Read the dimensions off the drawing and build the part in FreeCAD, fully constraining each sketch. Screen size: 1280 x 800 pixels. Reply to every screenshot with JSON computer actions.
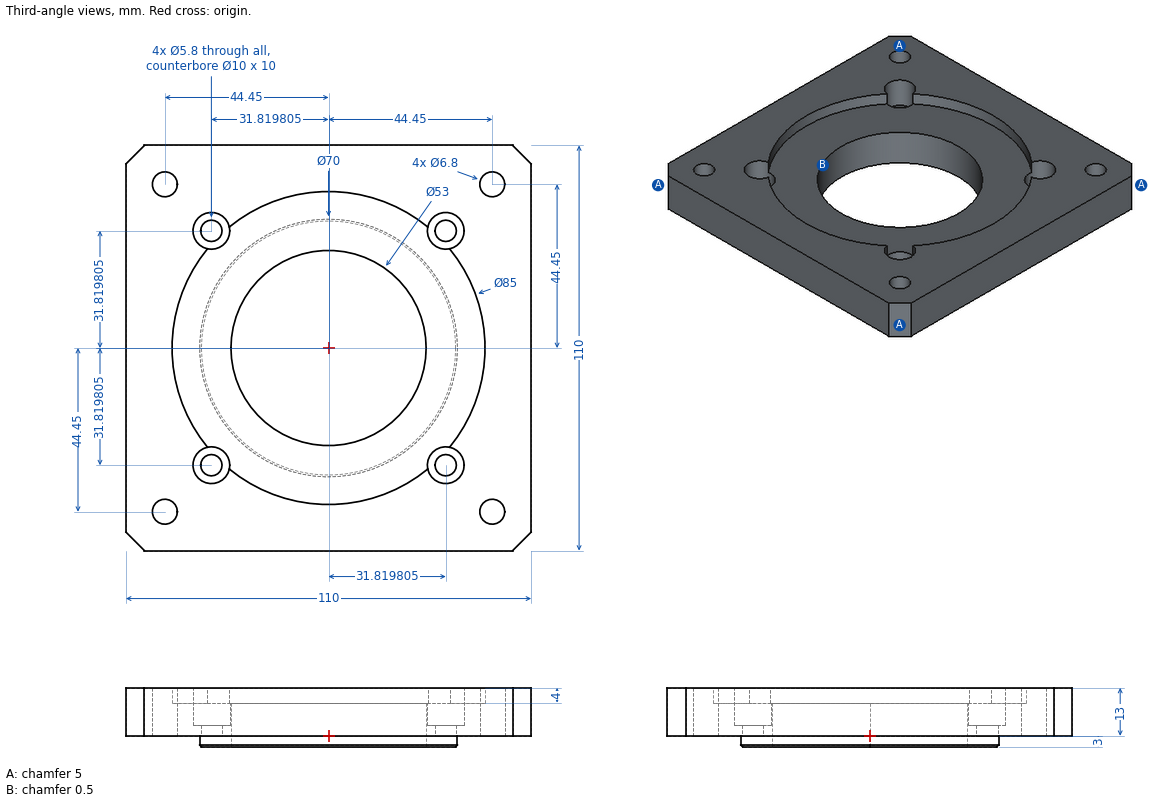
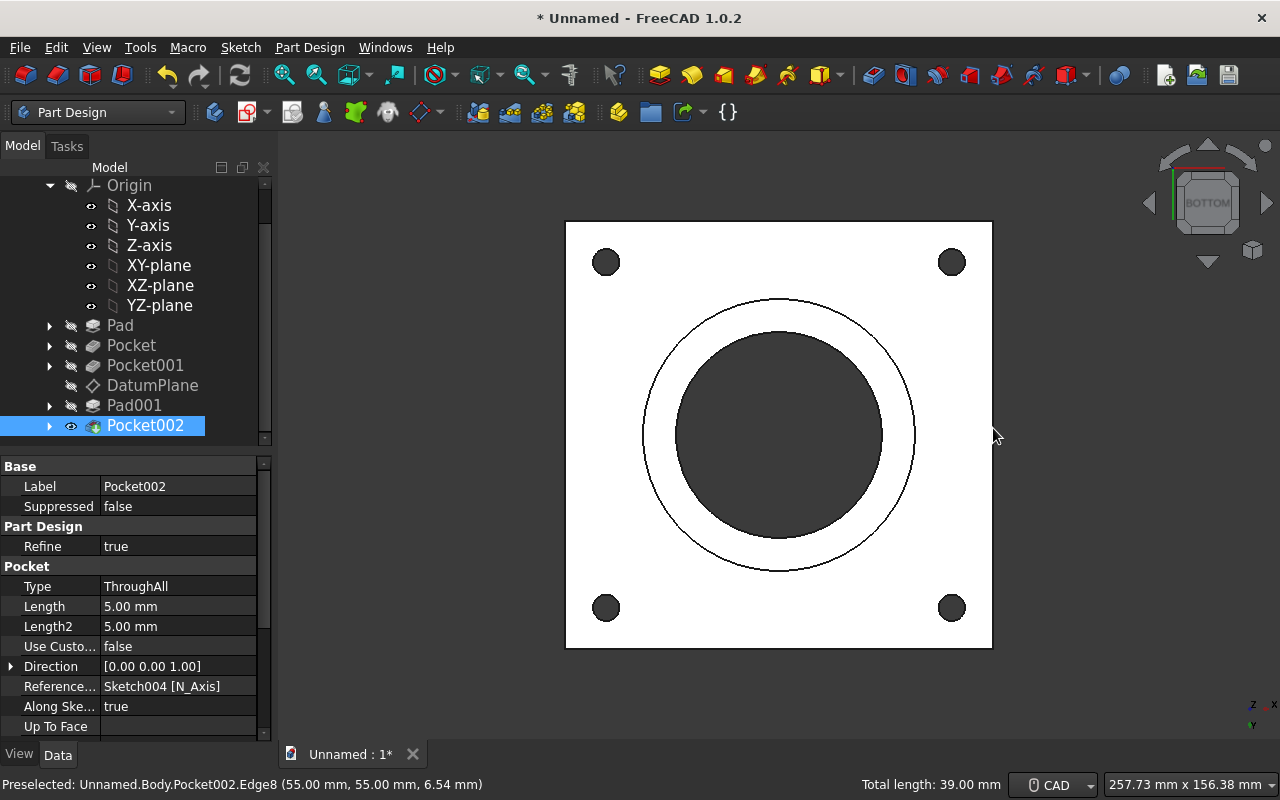
{"action": "key", "text": "4"}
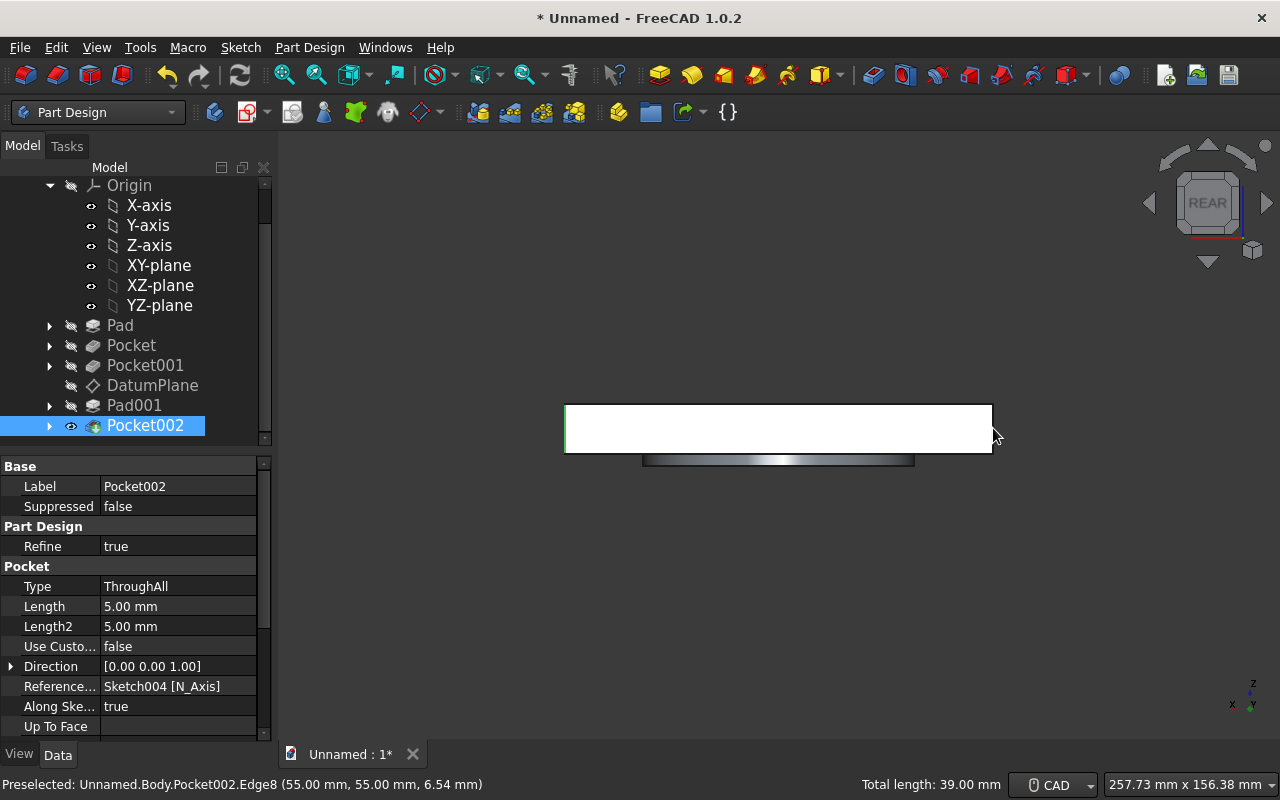
{"action": "left_click", "coordinate": [286, 76]}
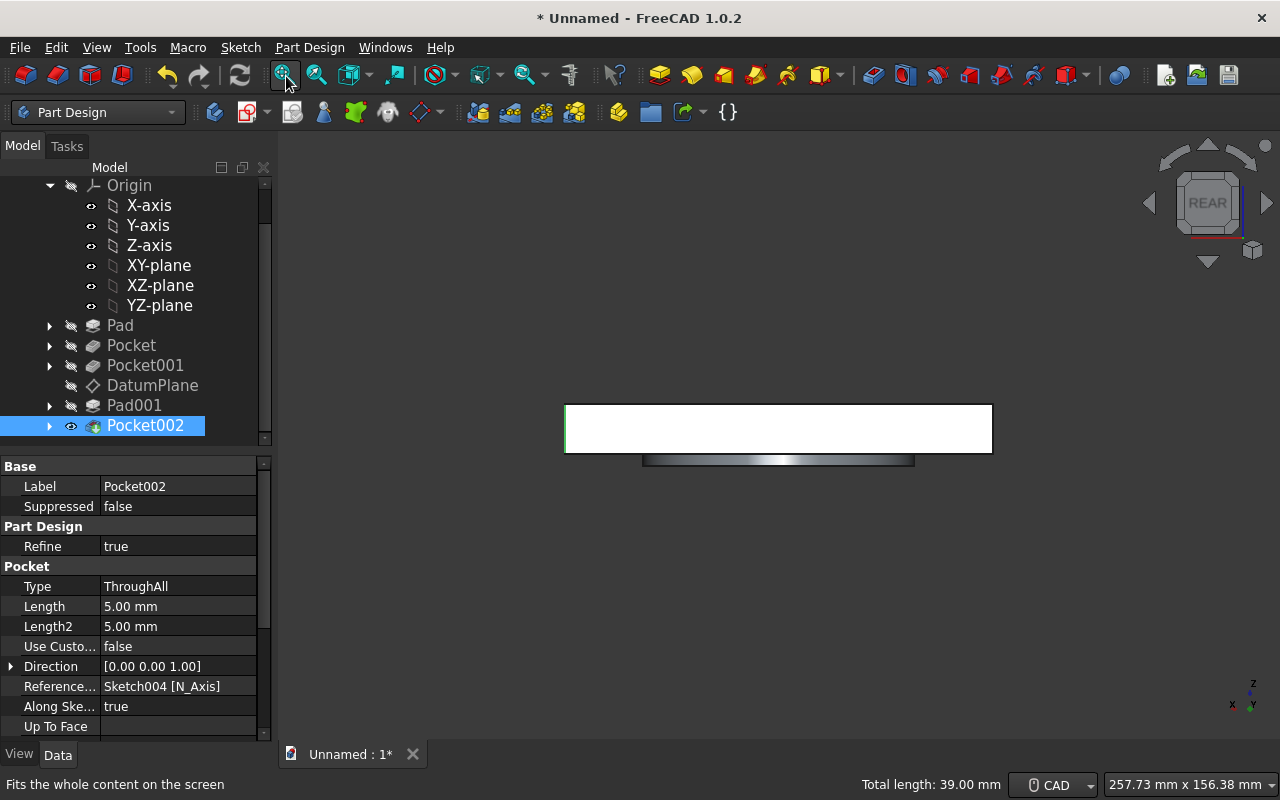
{"action": "left_click", "coordinate": [993, 428], "text": "ctrl"}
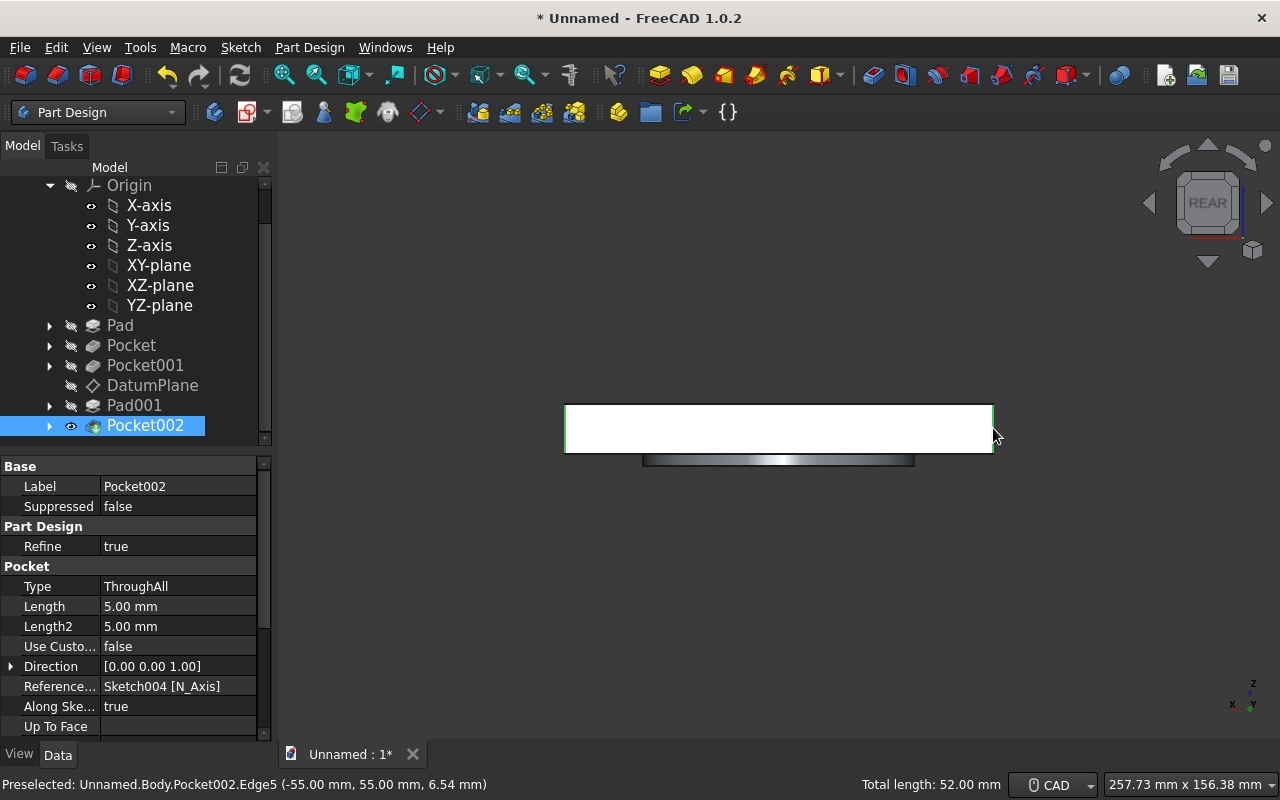
{"action": "left_click", "coordinate": [58, 76]}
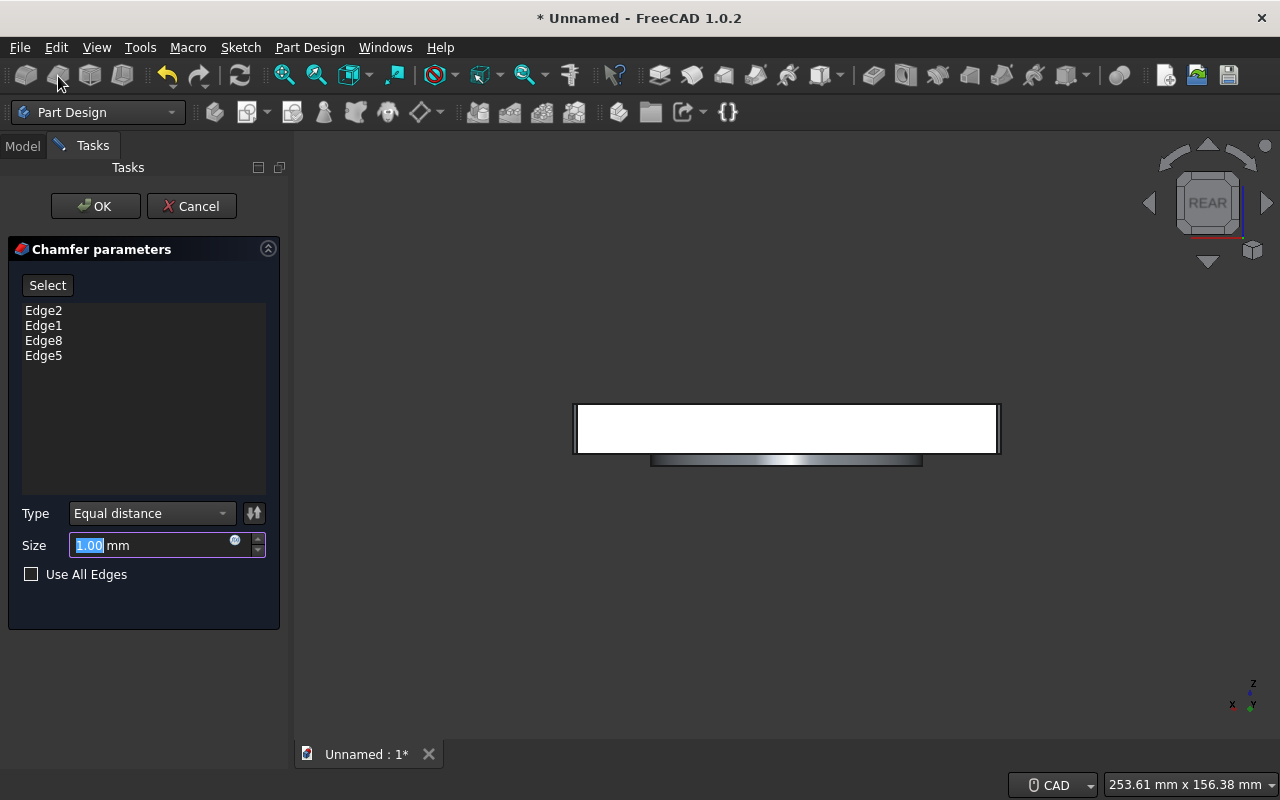
{"action": "type", "text": "5"}
{"action": "key", "text": "Tab"}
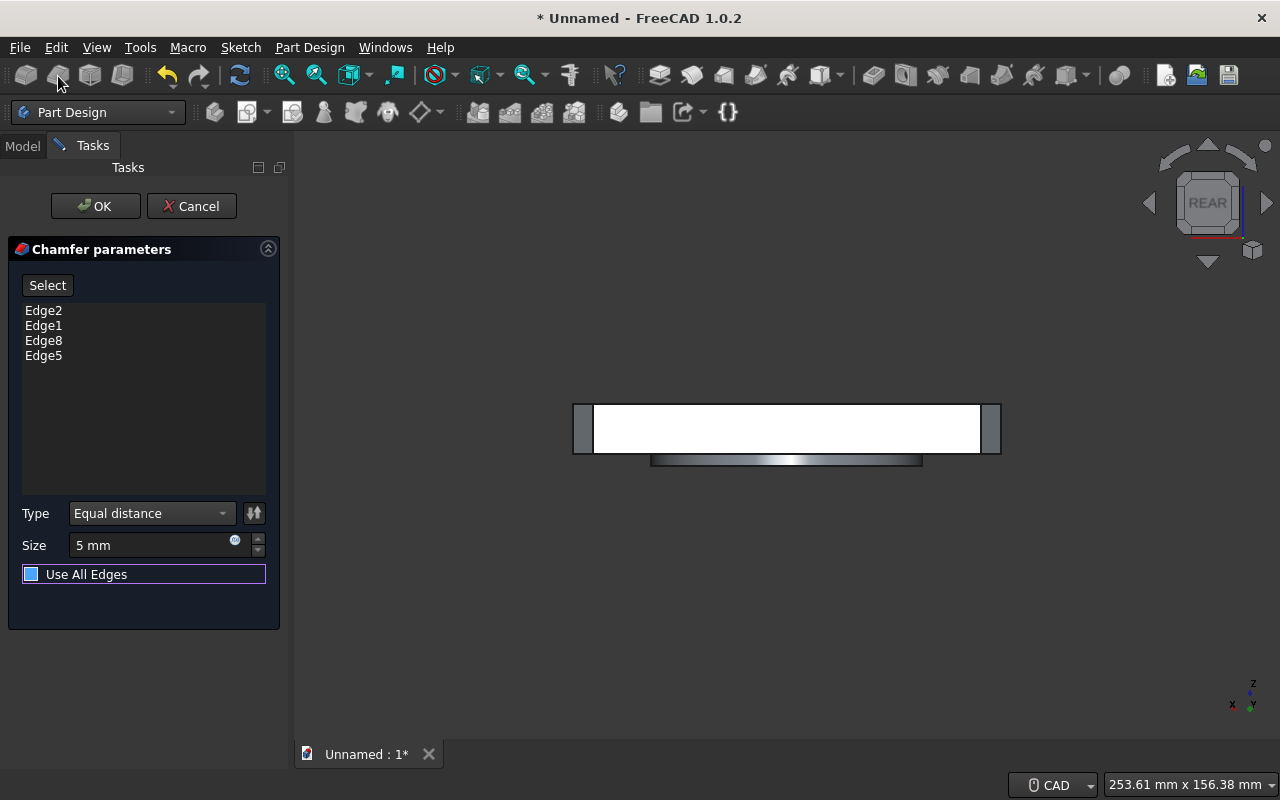
{"action": "left_click", "coordinate": [96, 206]}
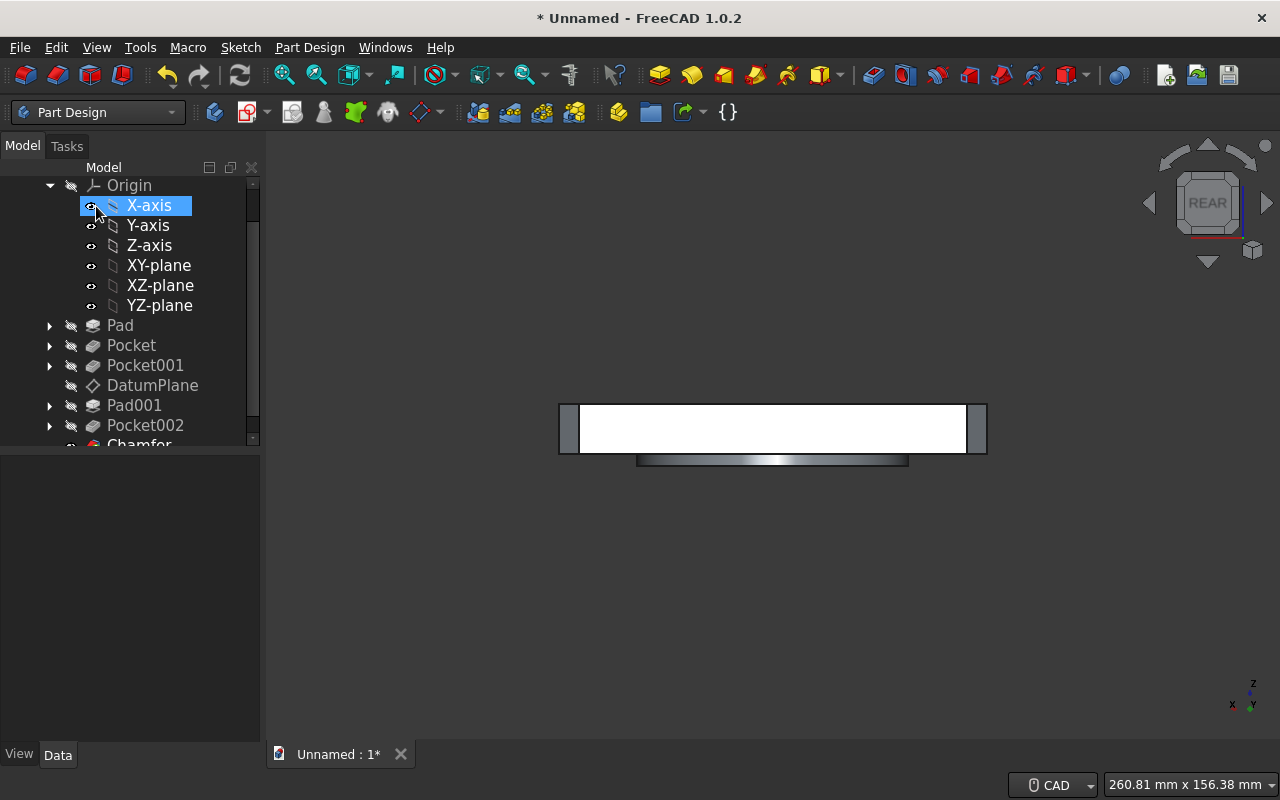
{"action": "key", "text": "v f"}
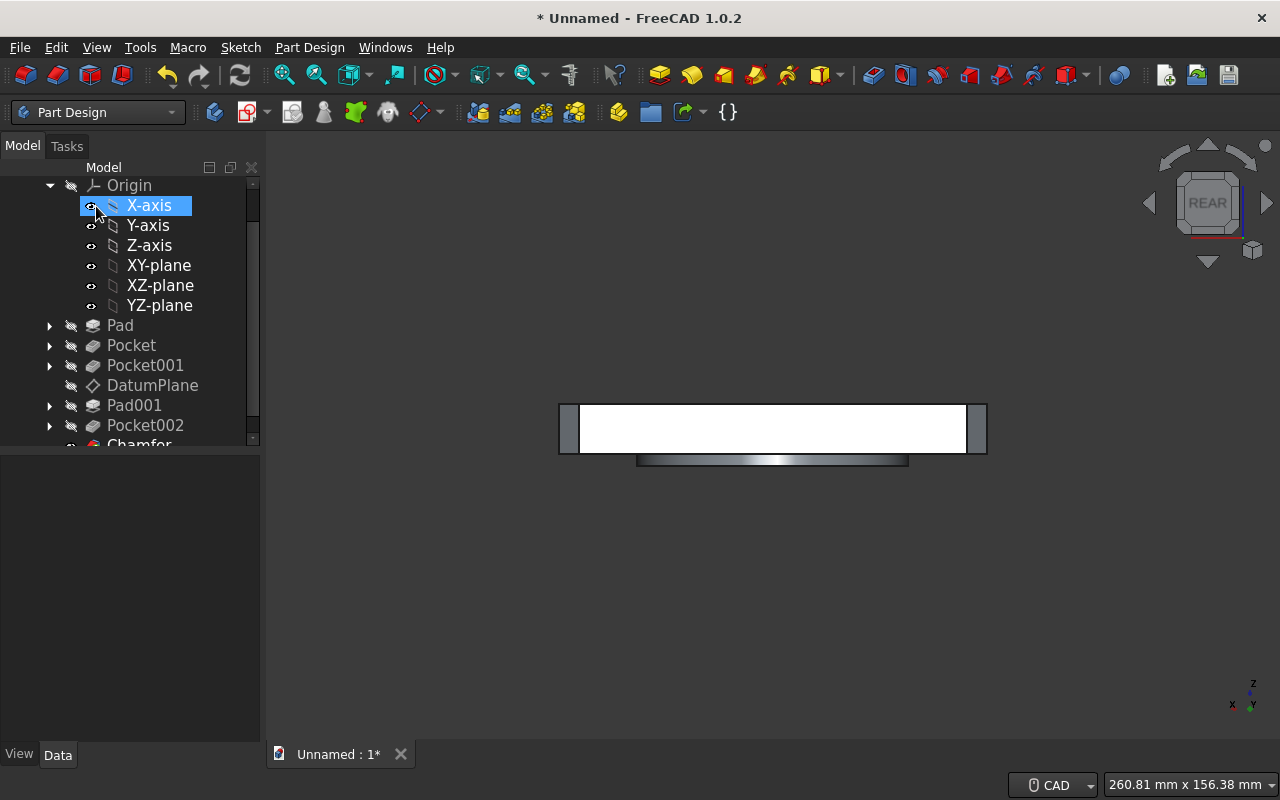
{"action": "key", "text": "0"}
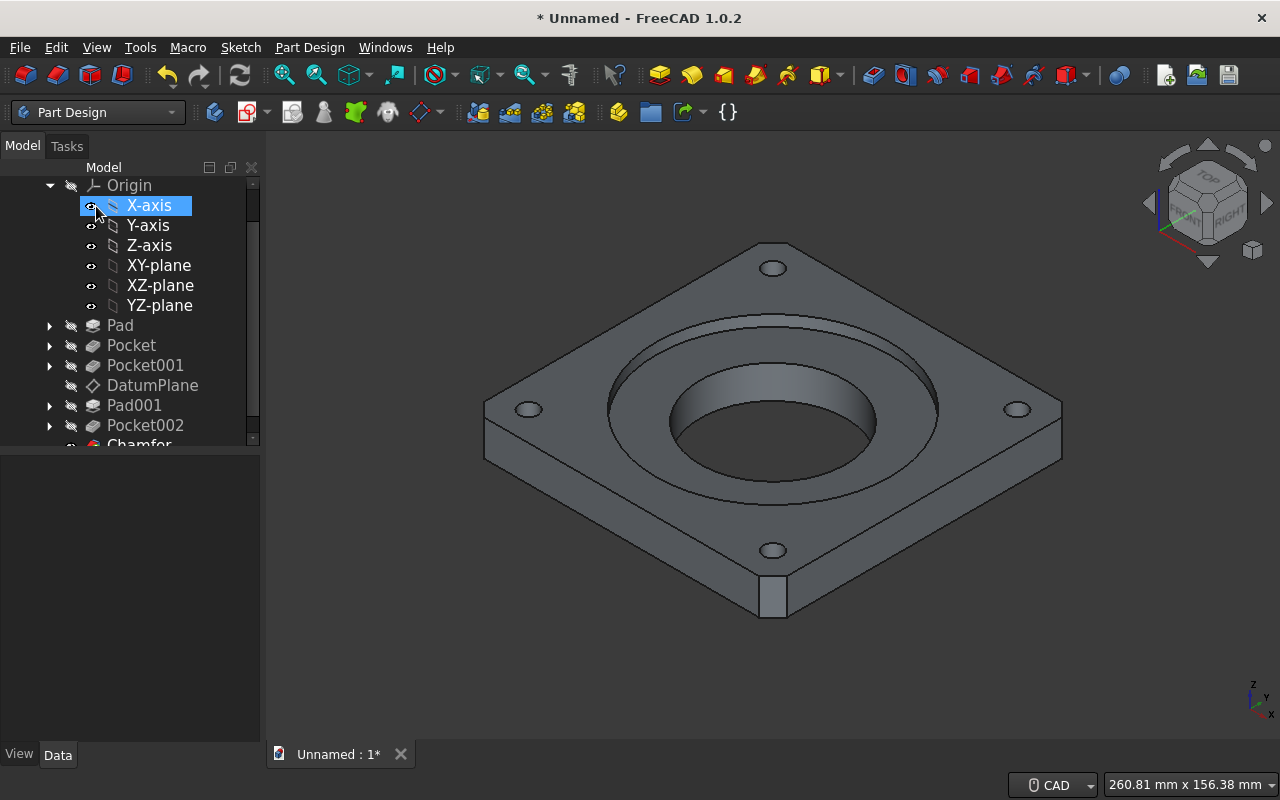
{"action": "left_click", "coordinate": [989, 434]}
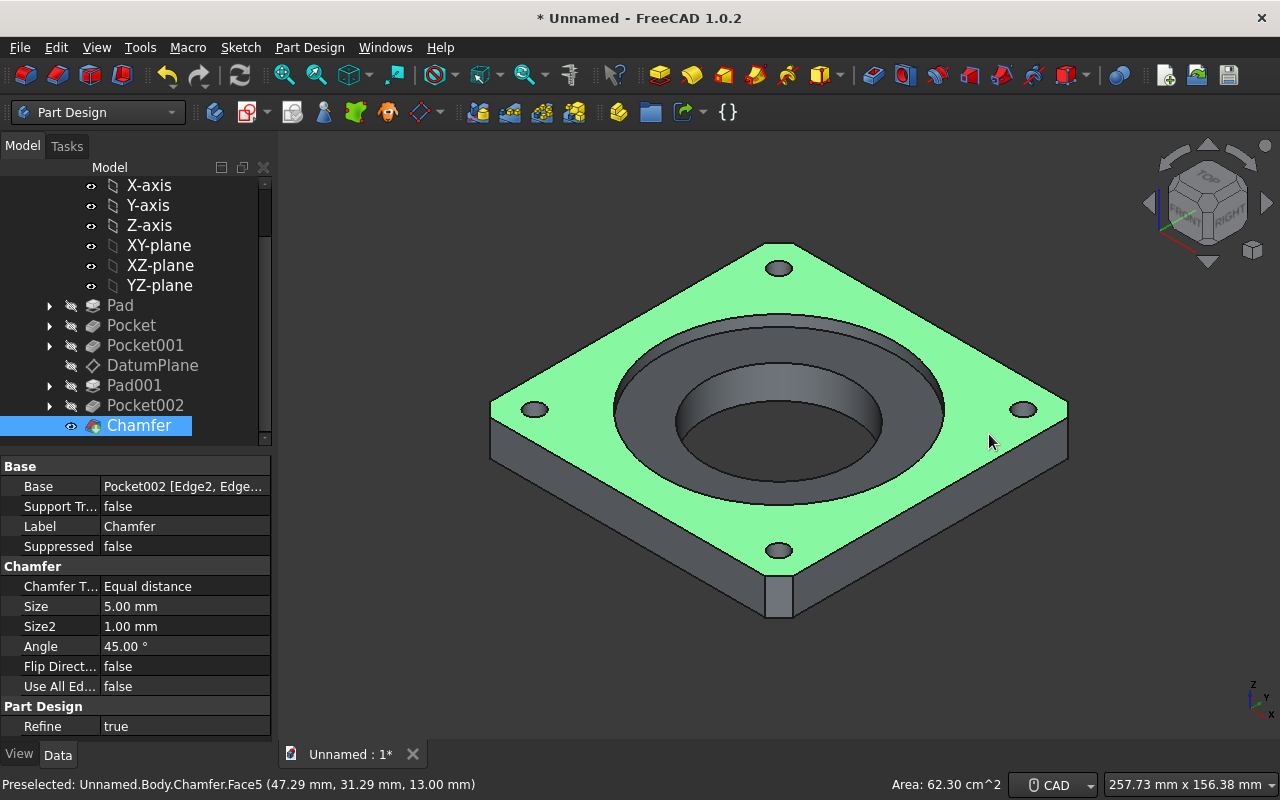
{"action": "left_click", "coordinate": [248, 112]}